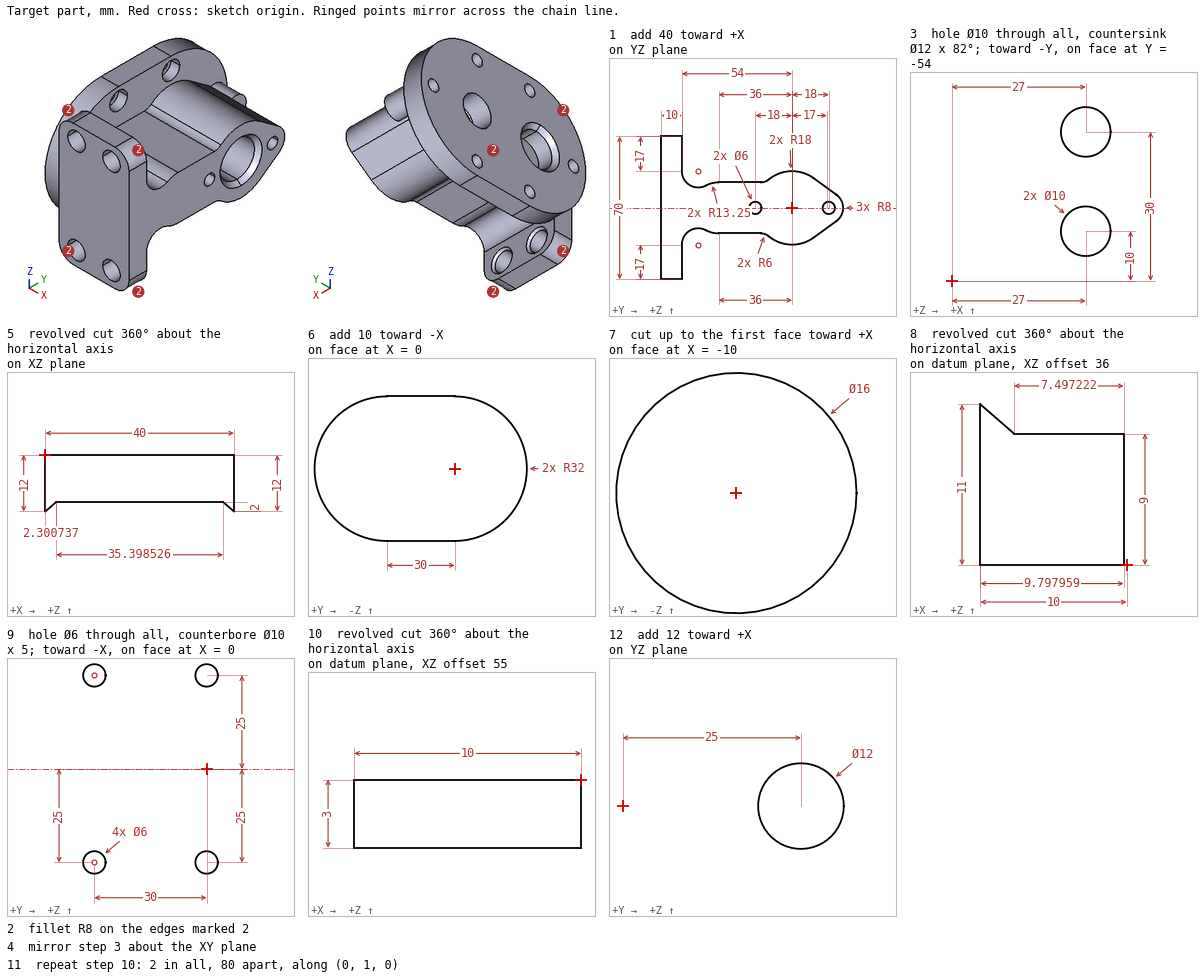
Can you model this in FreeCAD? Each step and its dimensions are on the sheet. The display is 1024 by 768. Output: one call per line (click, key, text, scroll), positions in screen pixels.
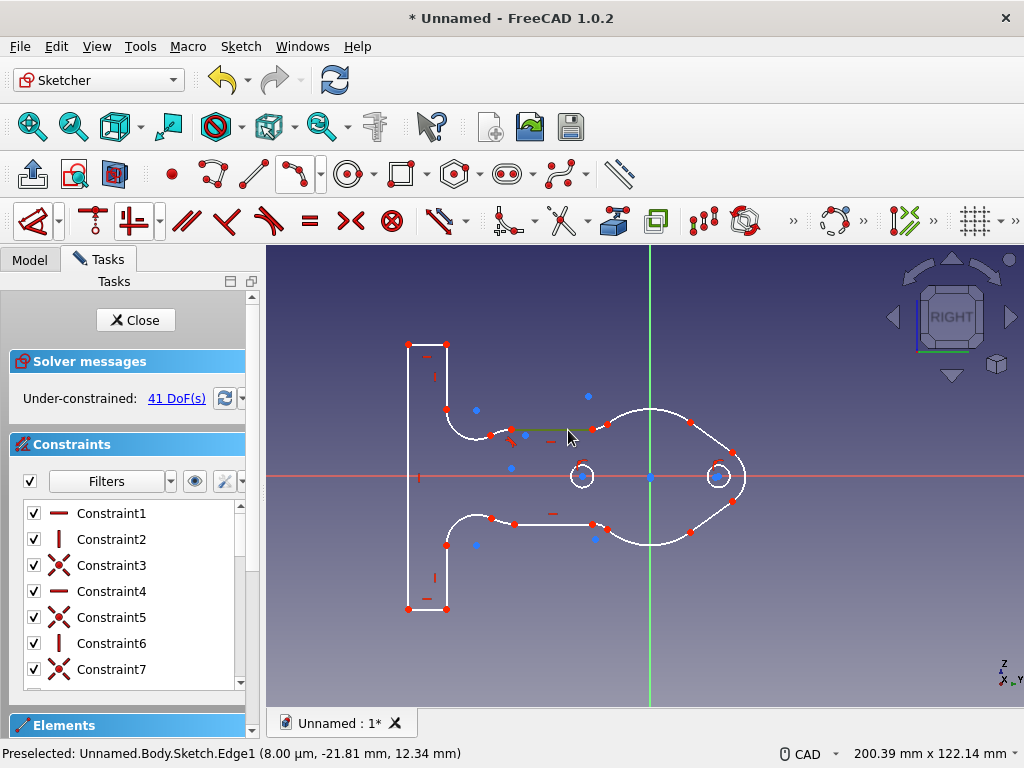
scroll(600, 428, up, 3)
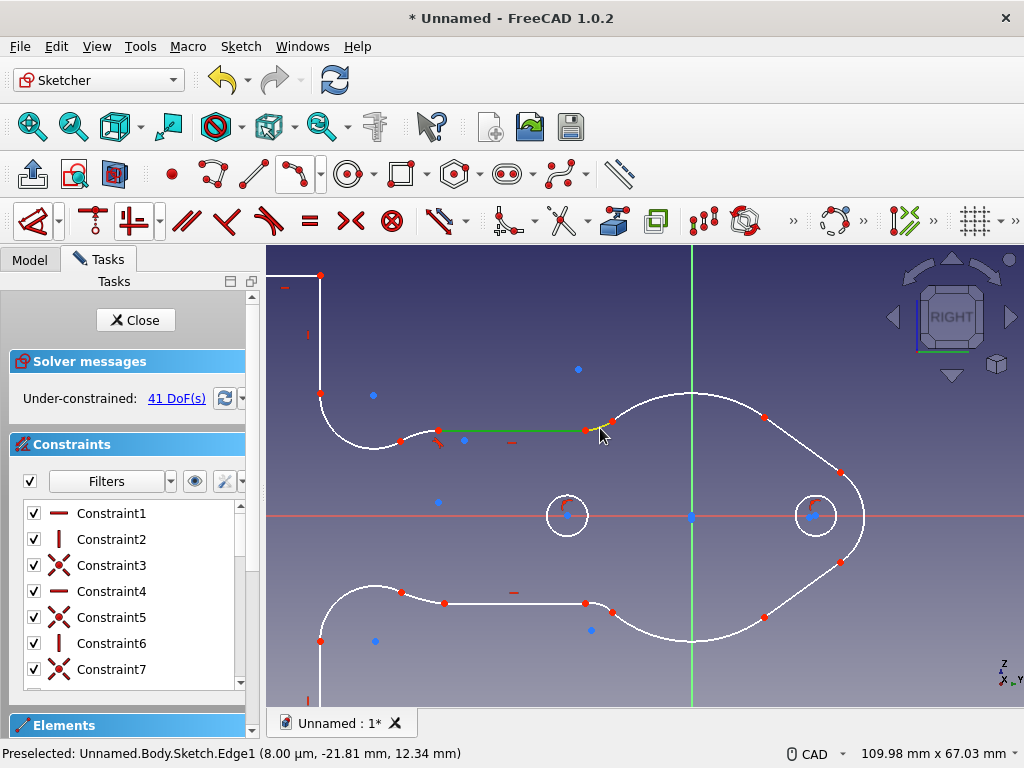
click(600, 427)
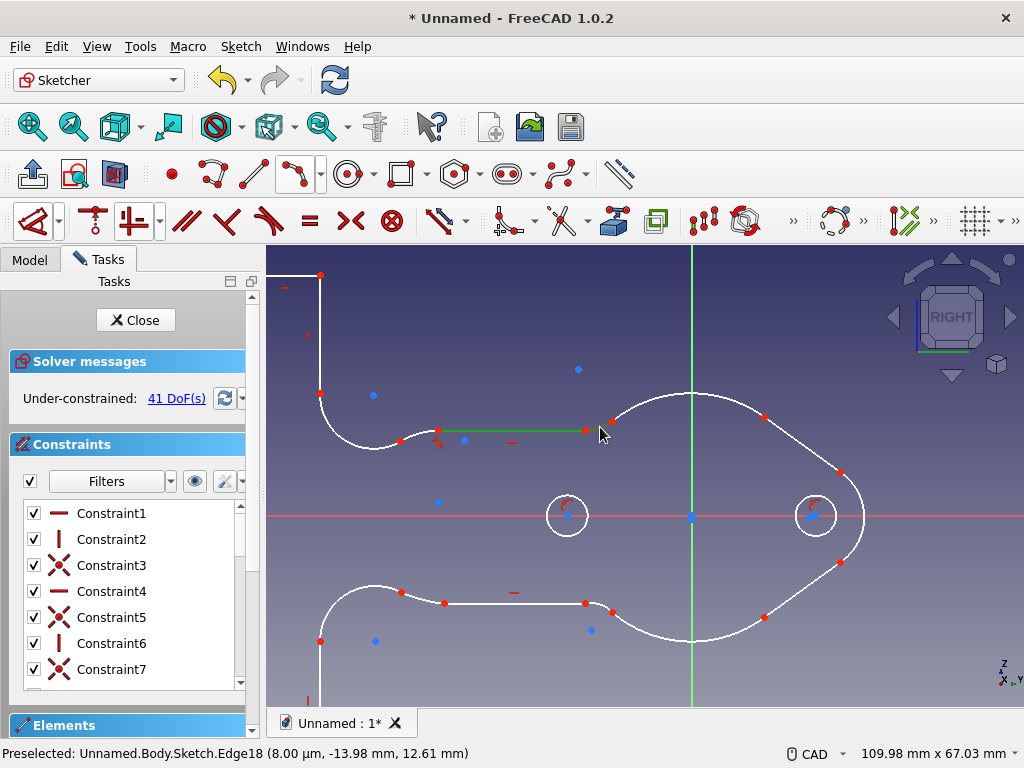
click(269, 222)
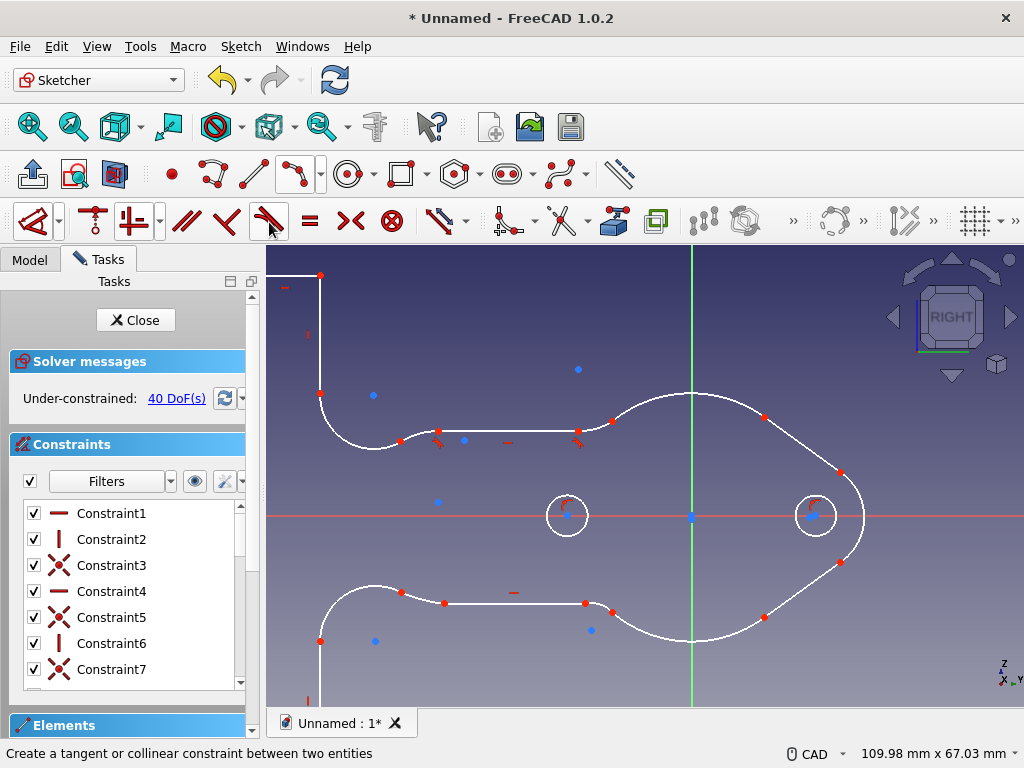
click(320, 358)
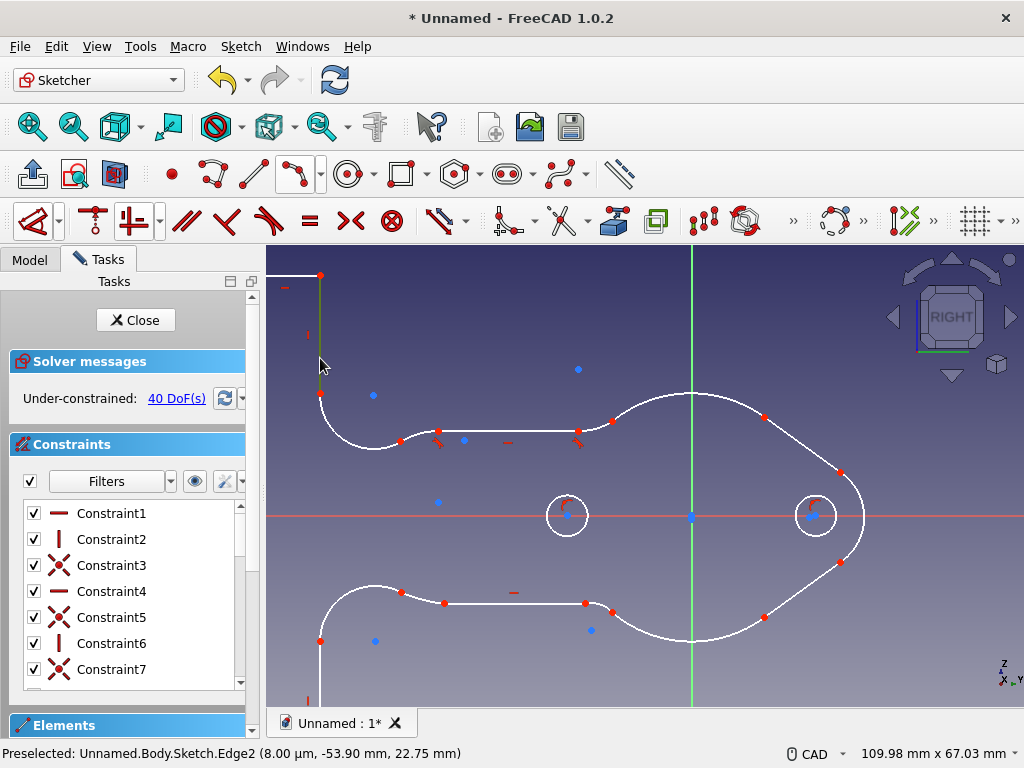
click(330, 426)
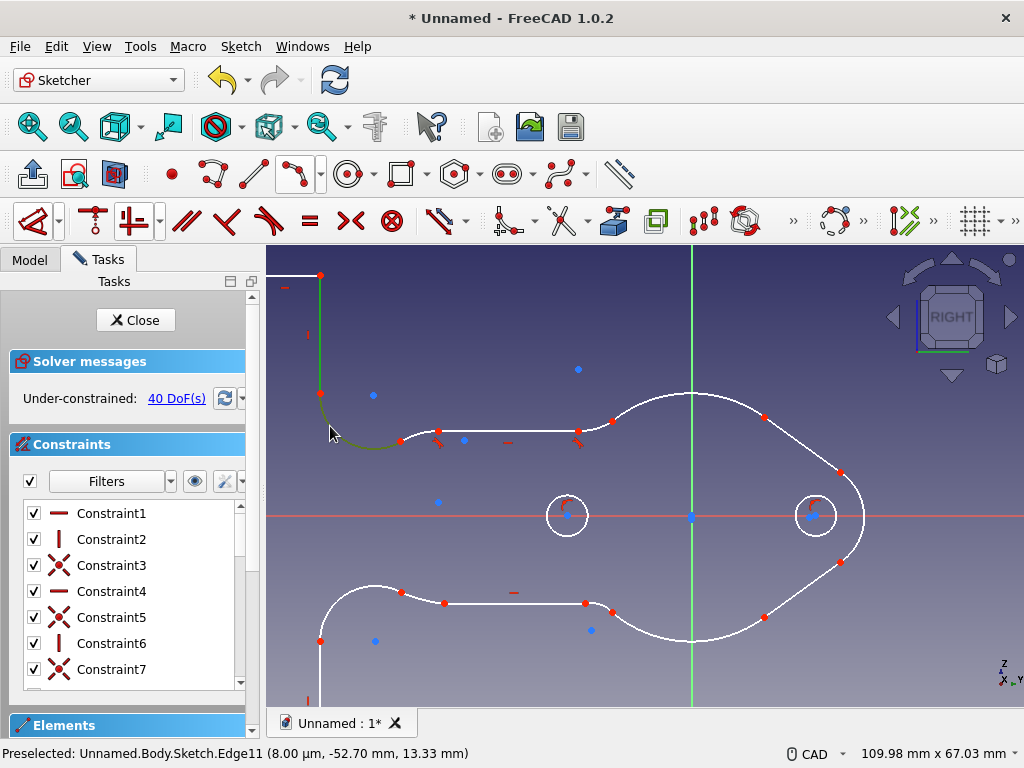
click(269, 222)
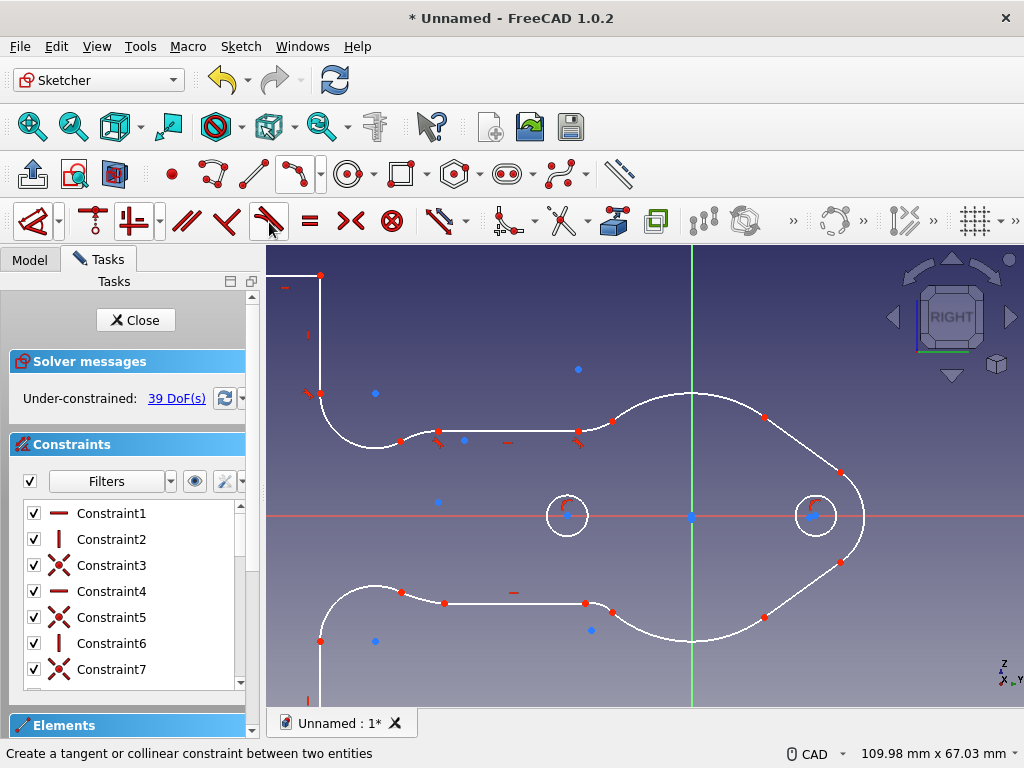
click(320, 676)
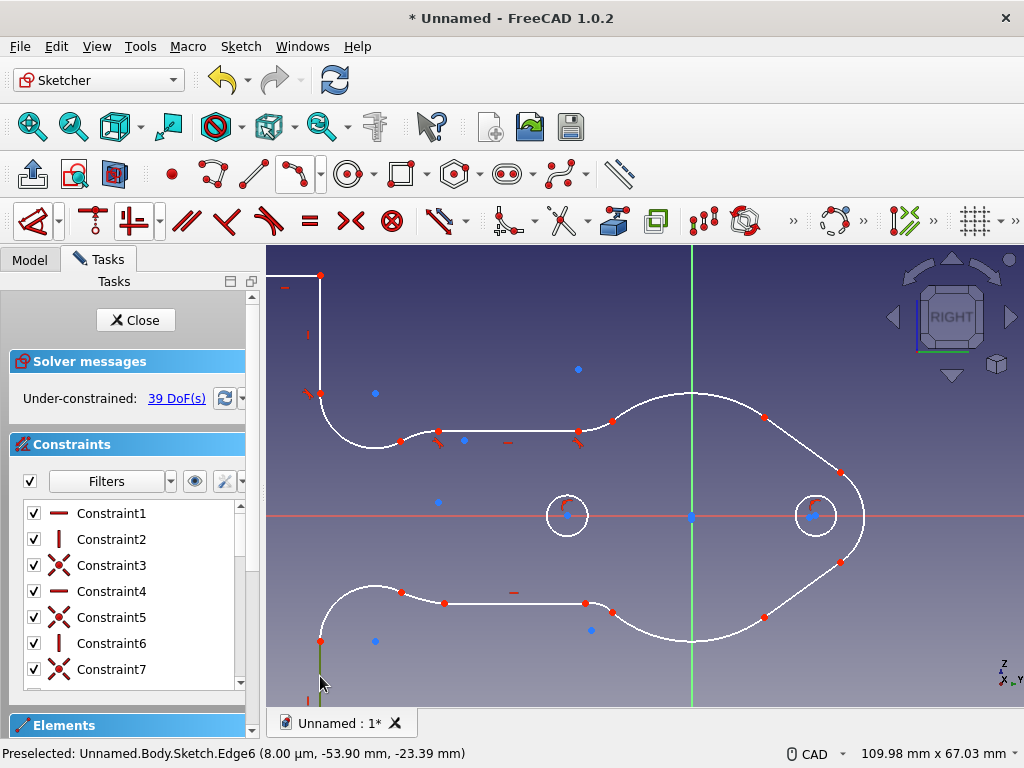
click(368, 587)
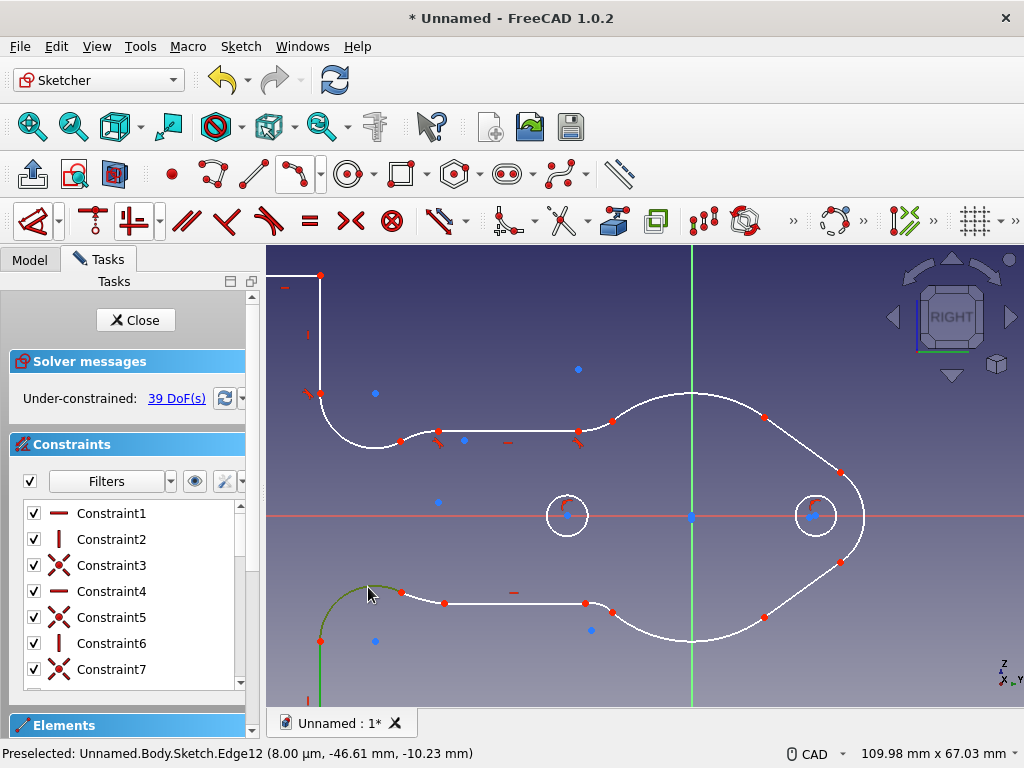
click(269, 222)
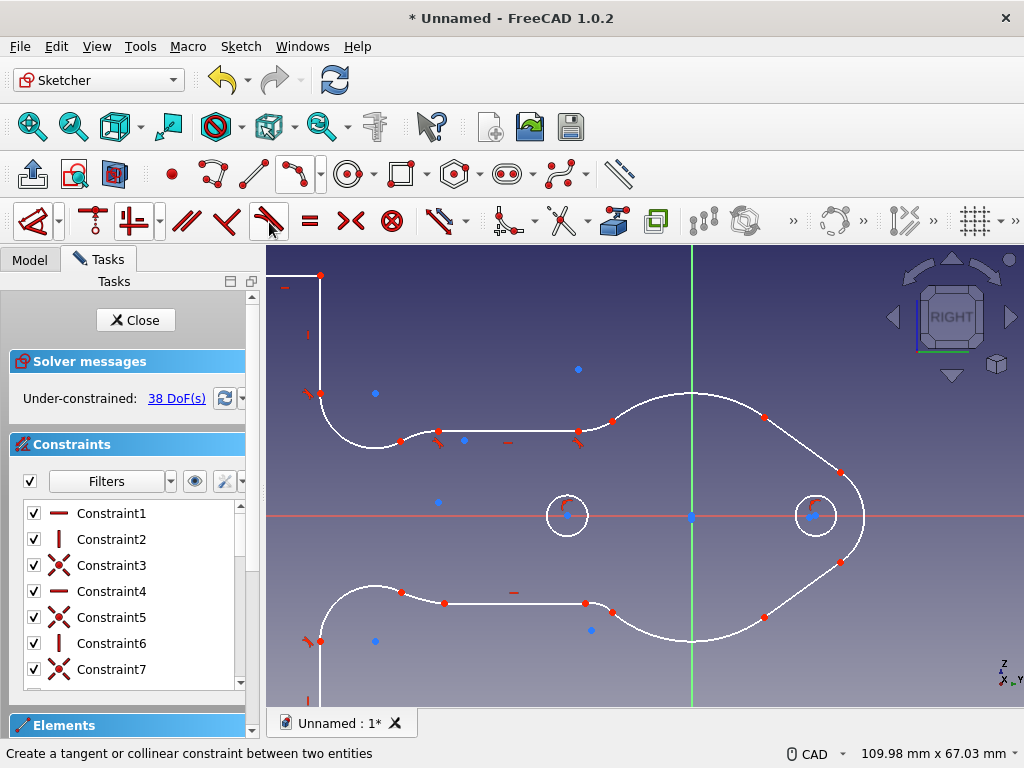
click(487, 604)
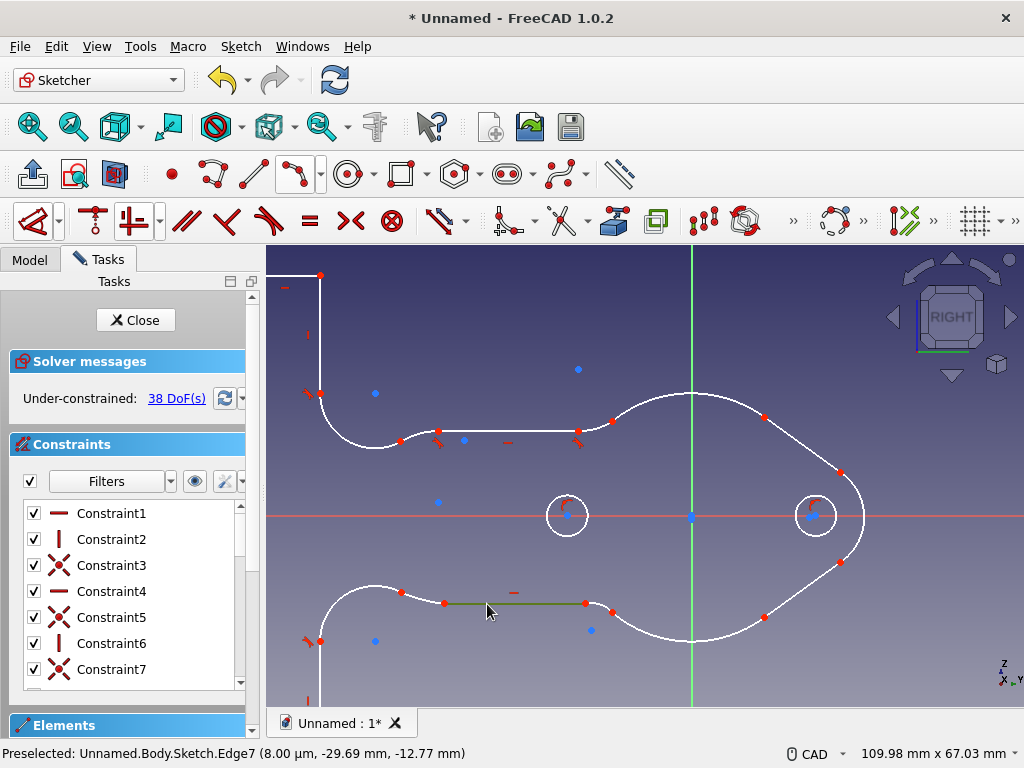
click(414, 597)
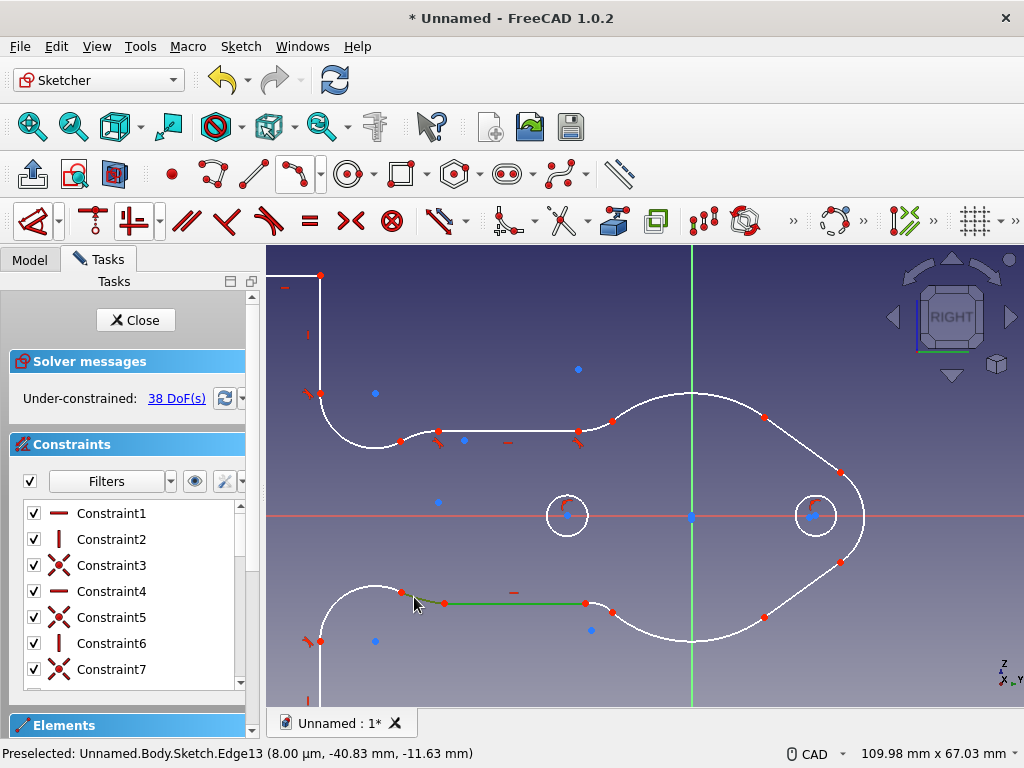
click(269, 222)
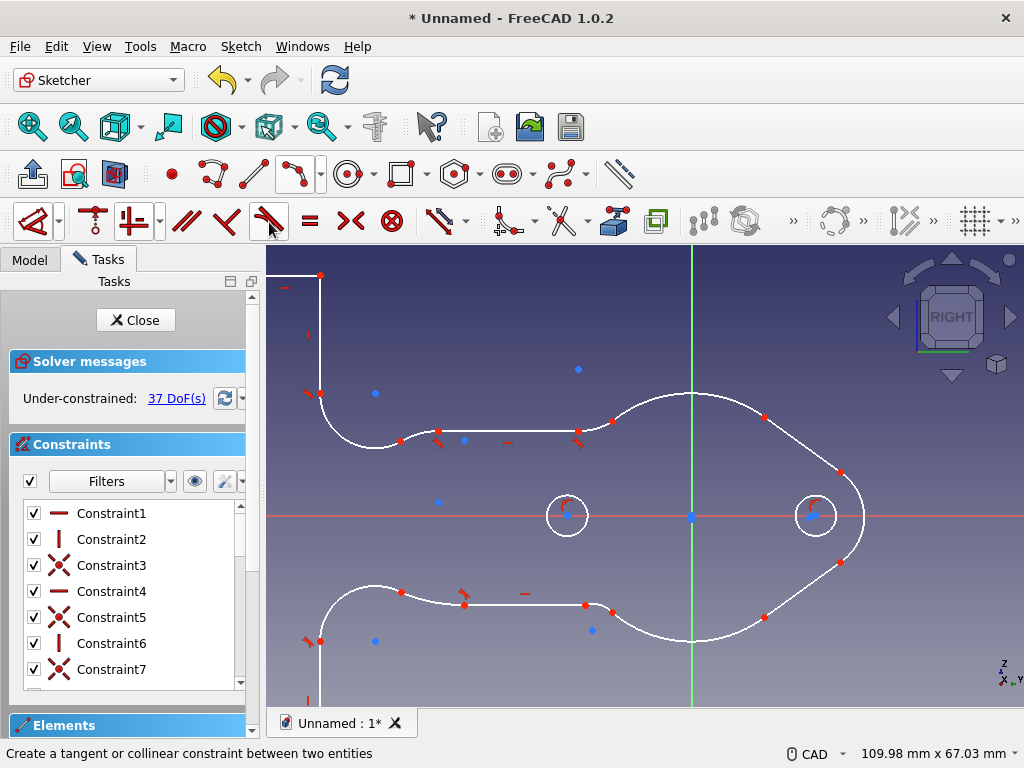
click(501, 605)